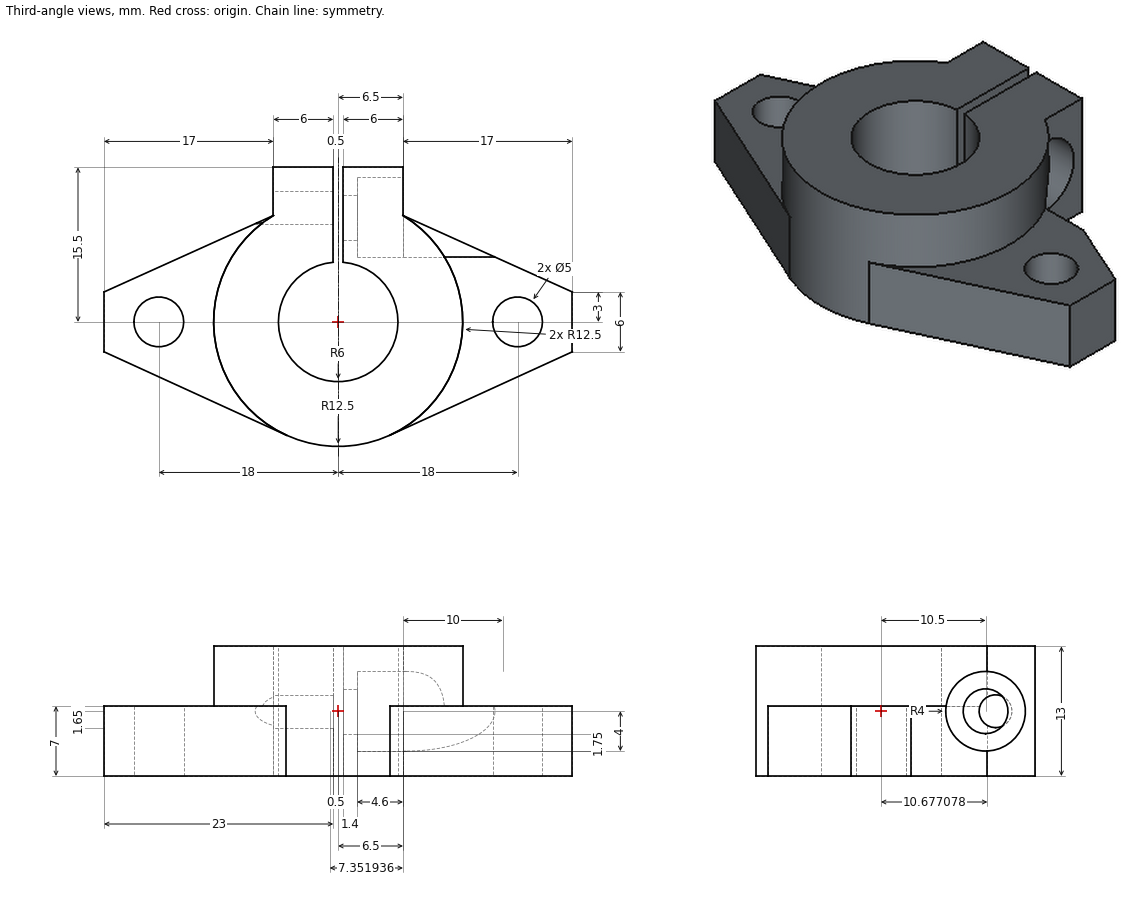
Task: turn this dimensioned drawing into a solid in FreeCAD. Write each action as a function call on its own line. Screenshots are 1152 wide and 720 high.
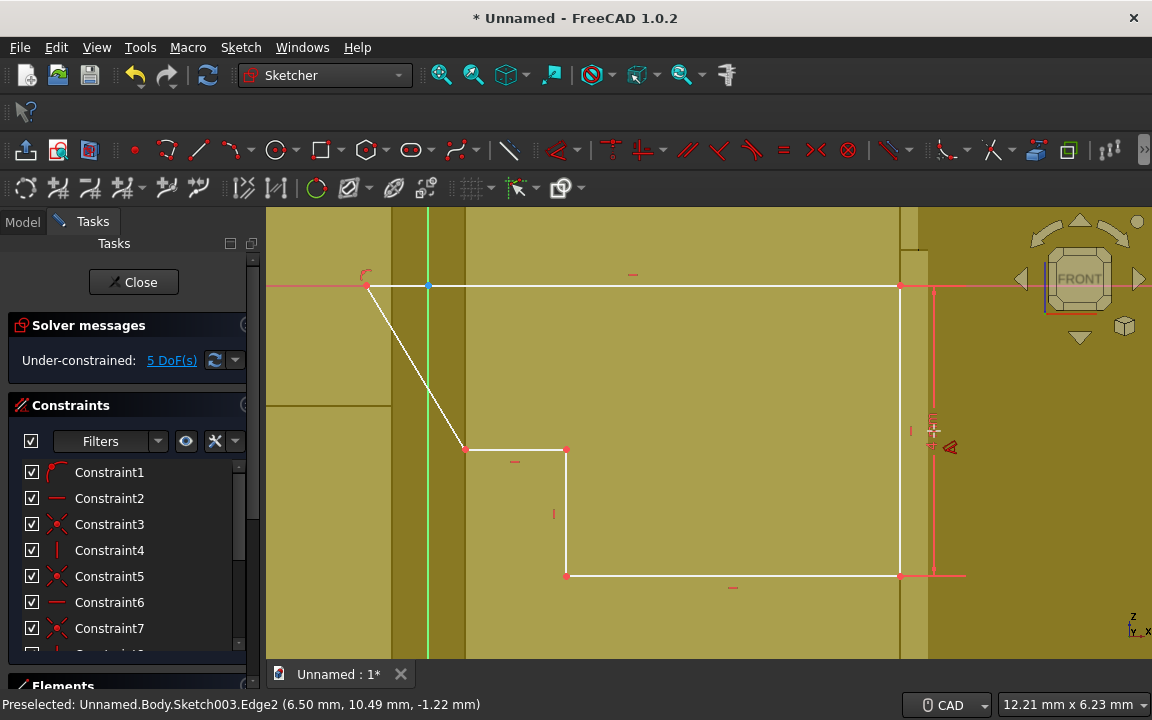
click(800, 576)
click(733, 610)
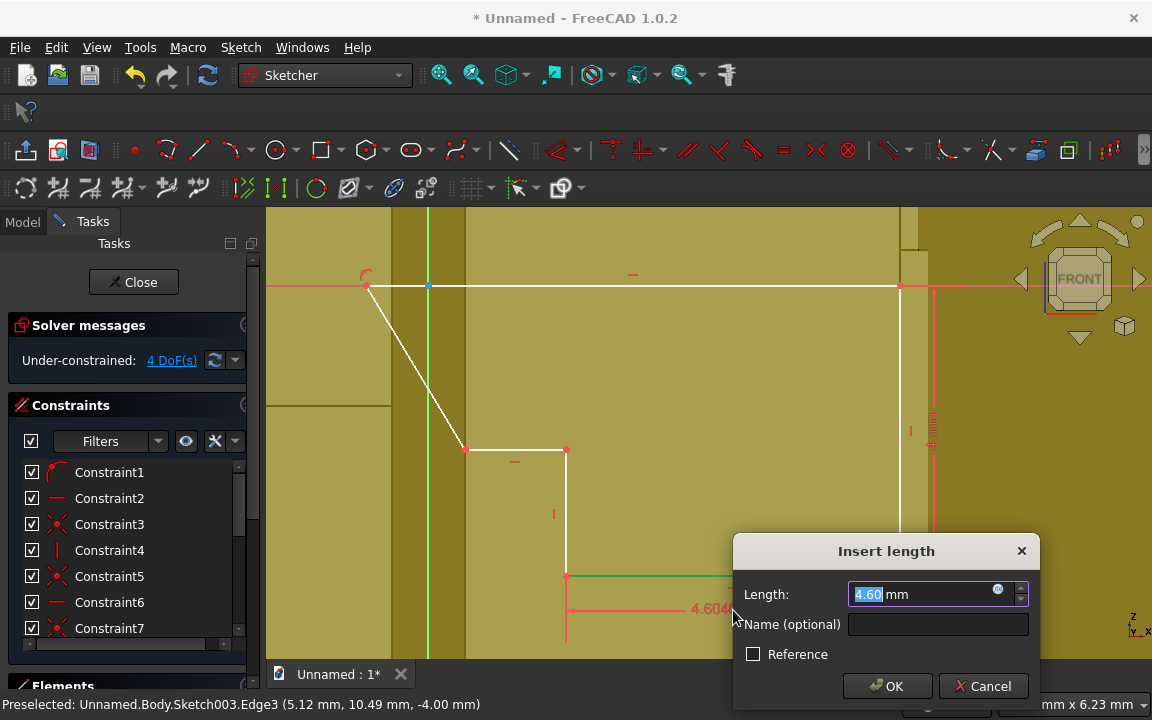
text(4.6)
key(Return)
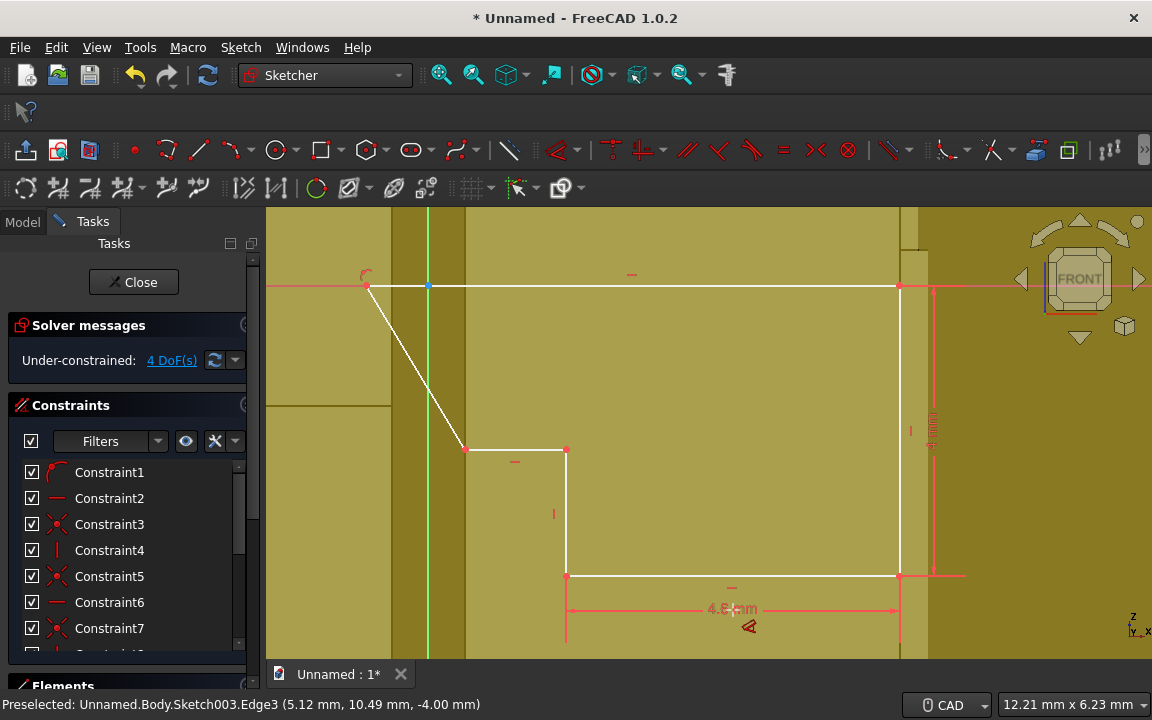
click(536, 450)
click(516, 484)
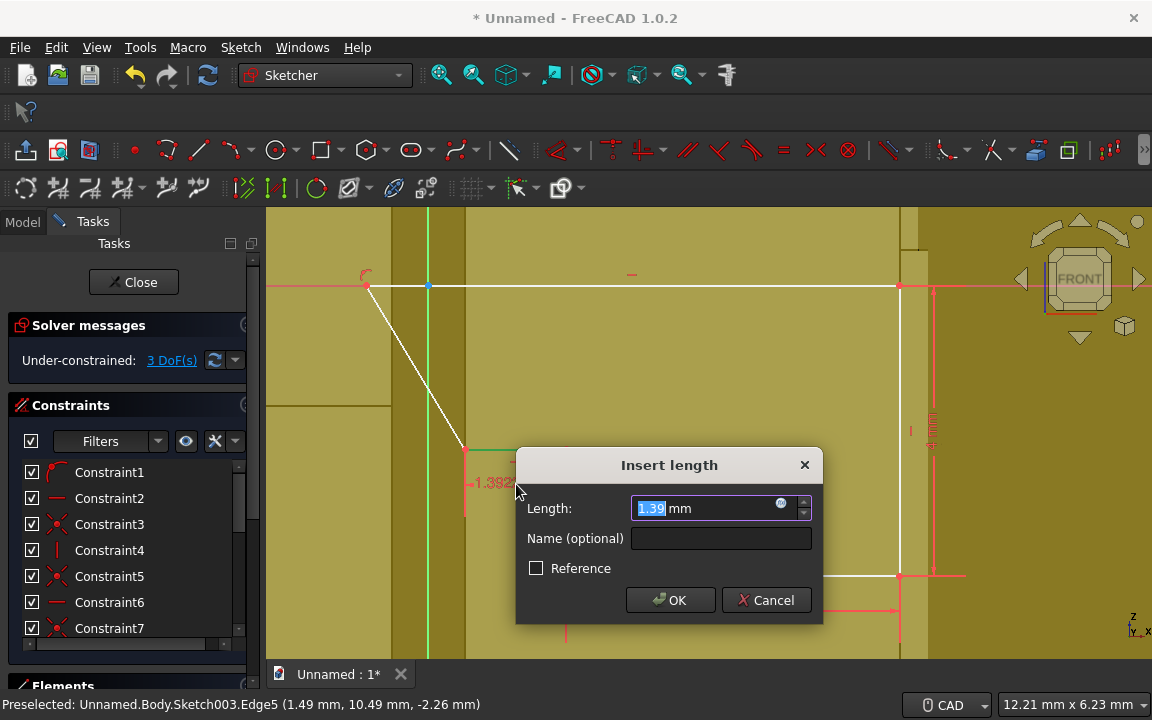
text(1.4)
key(Return)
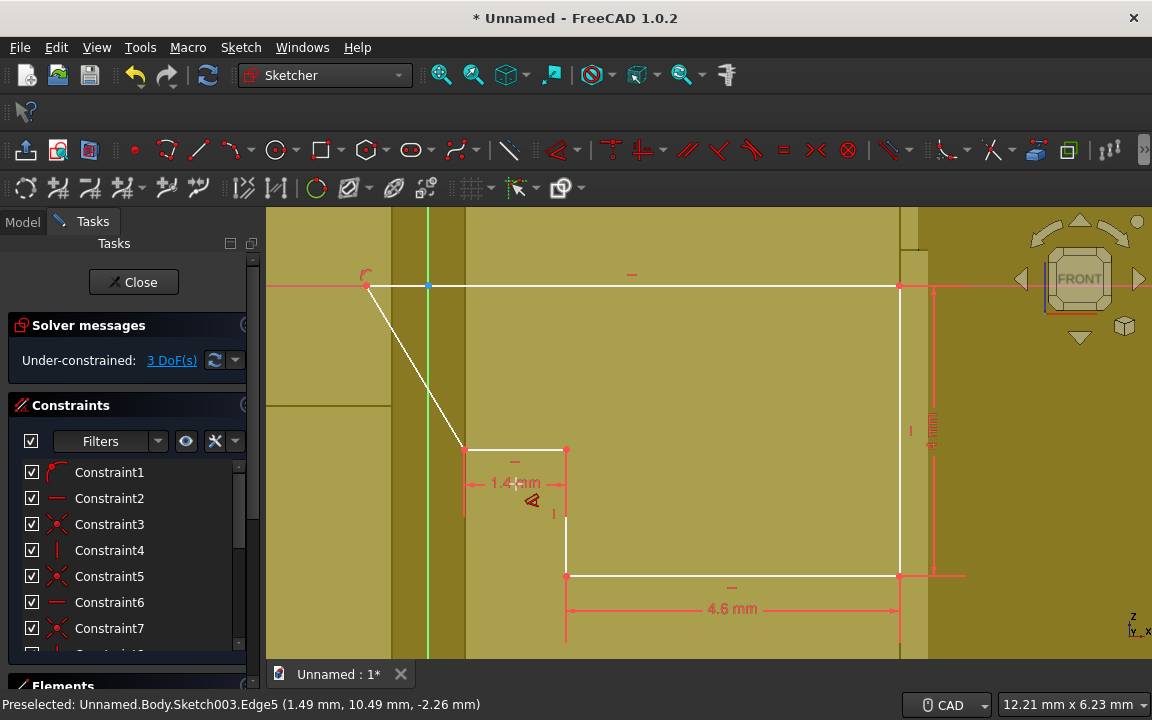
click(566, 538)
click(532, 513)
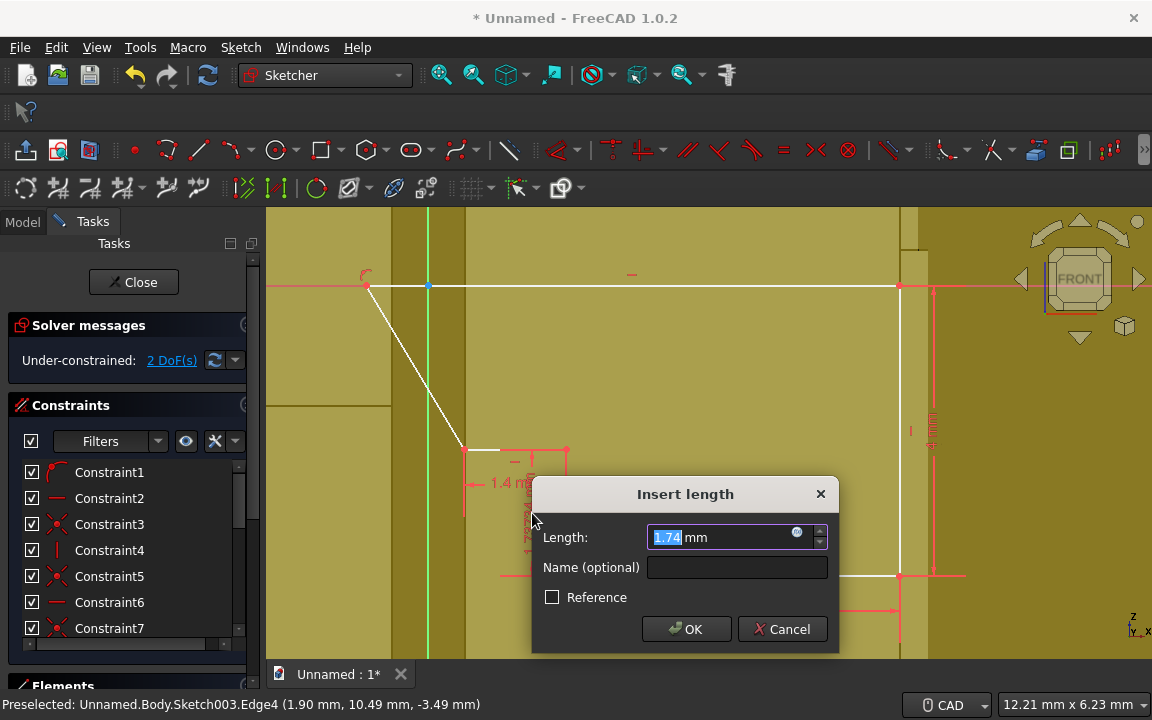
text(1.75)
key(Return)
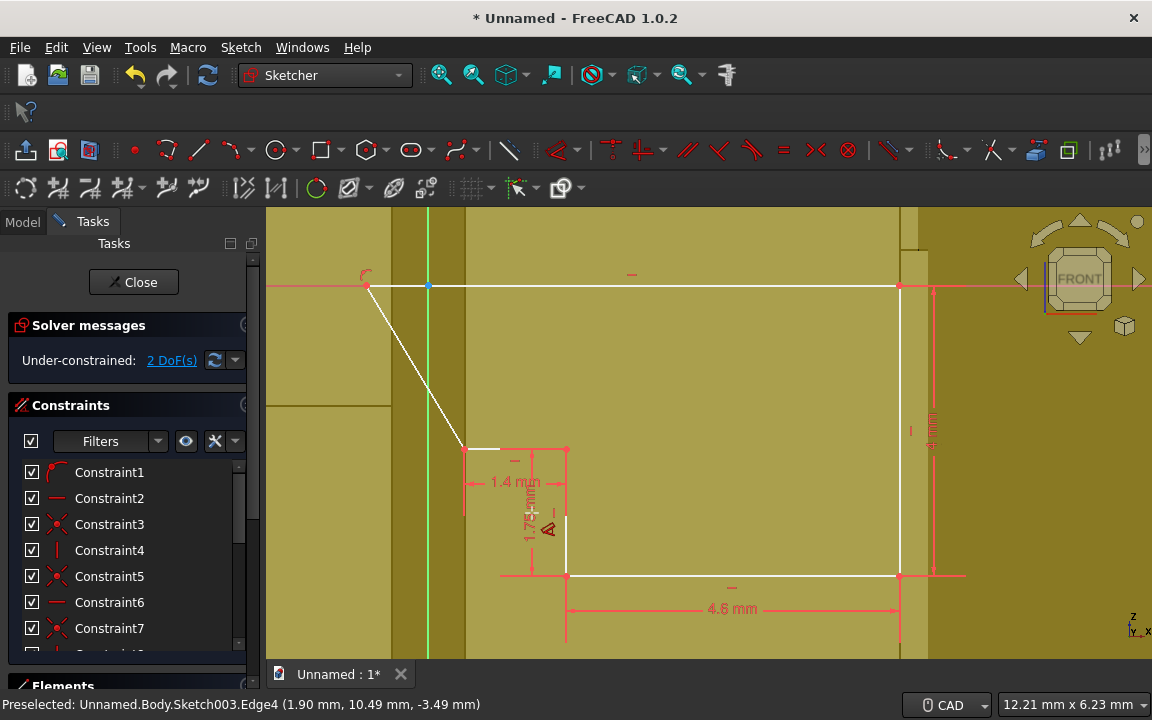
click(900, 286)
click(664, 252)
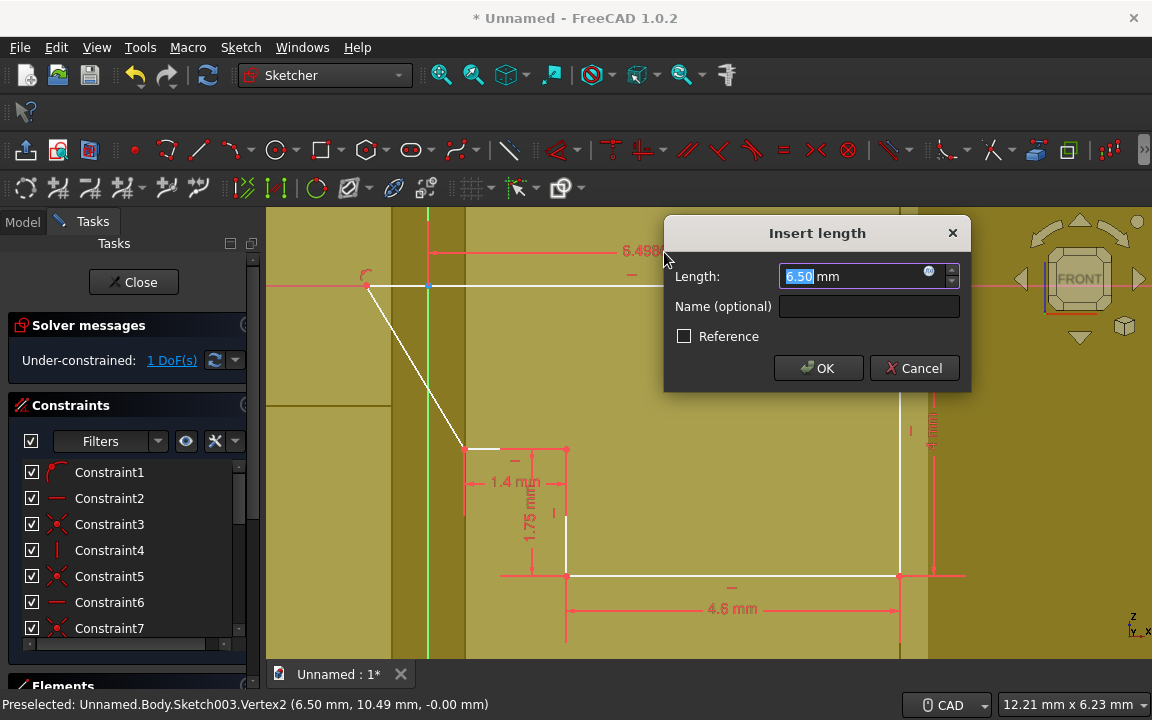
text(6.5)
key(Return)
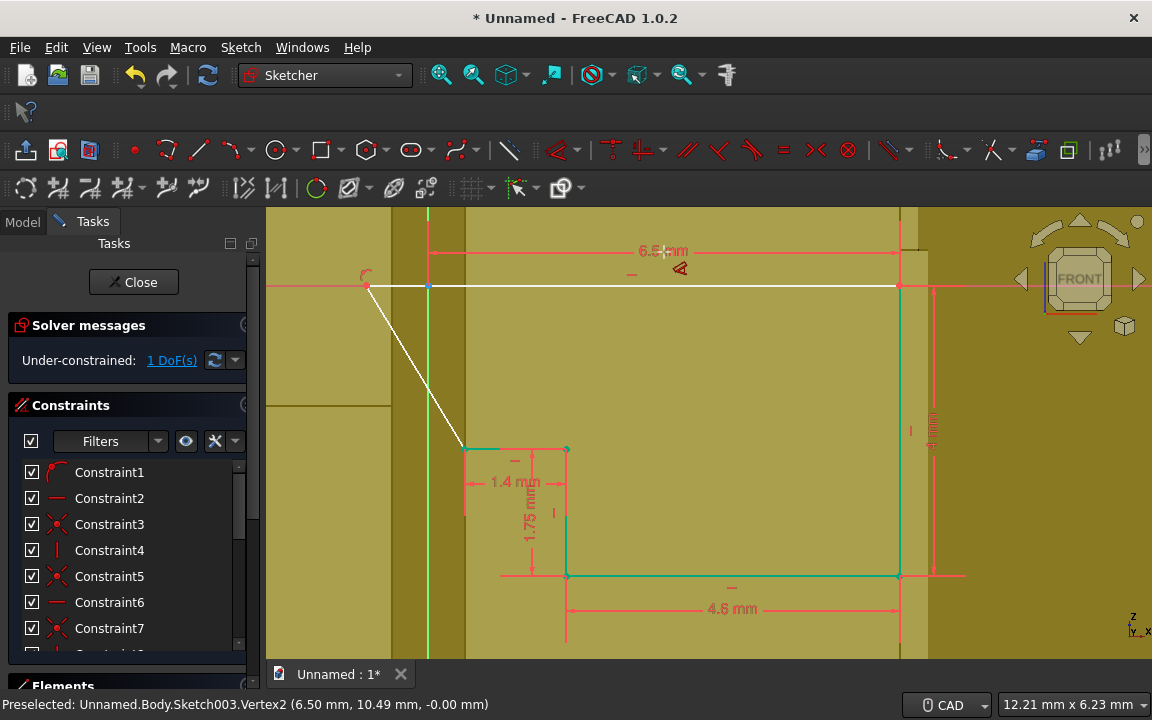
click(526, 286)
click(510, 252)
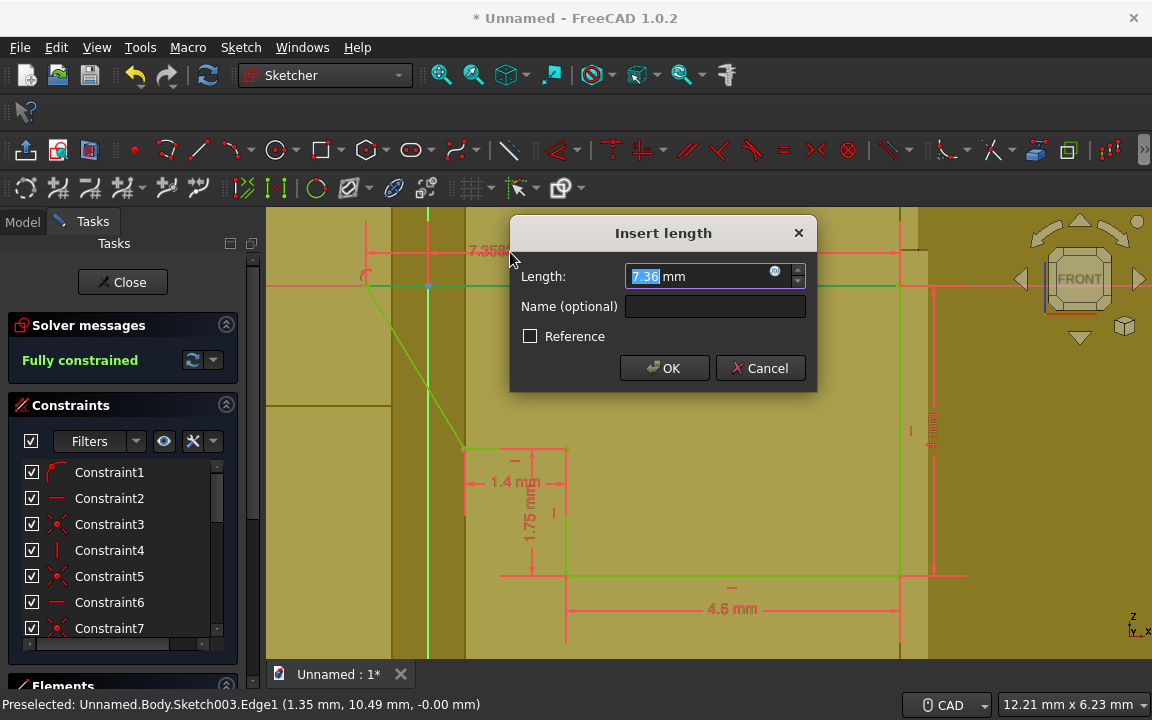
text(7.351936)
key(Return)
key(Escape)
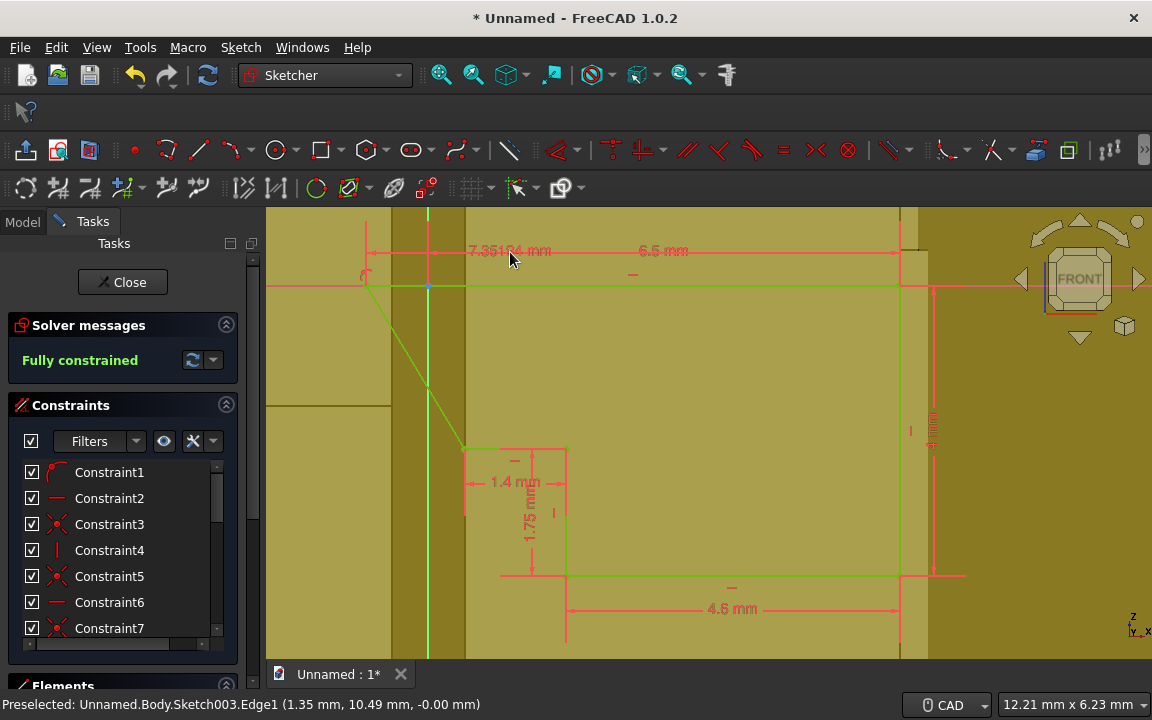
click(123, 282)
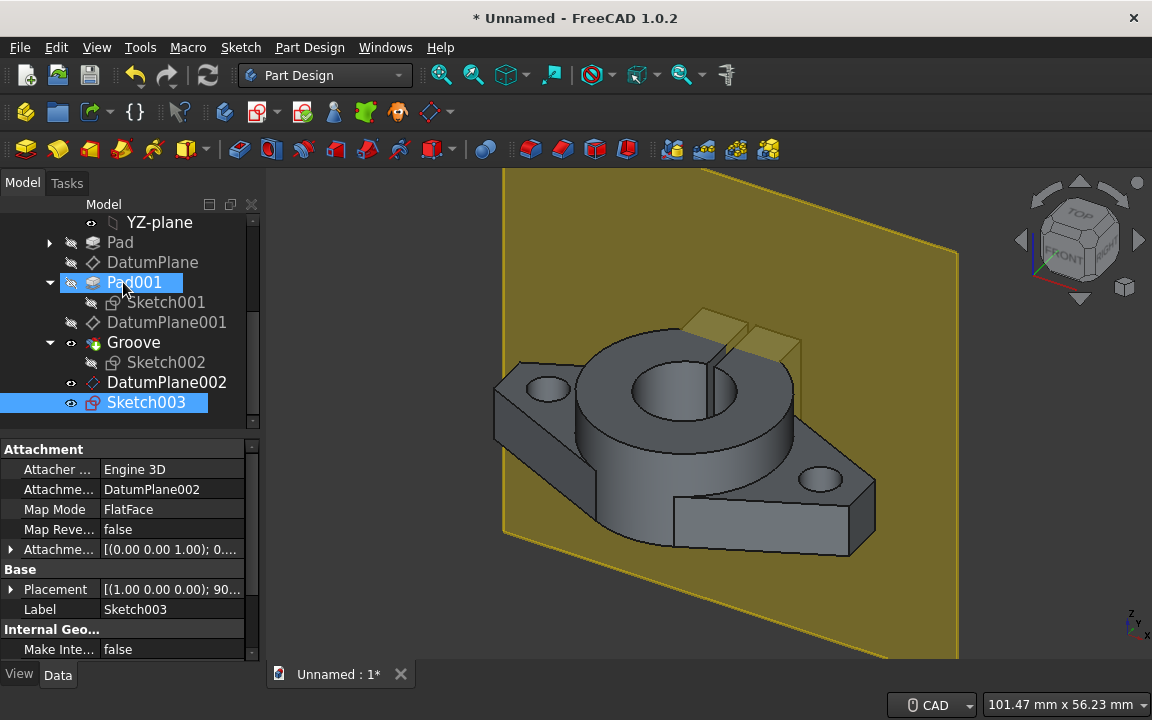
click(304, 150)